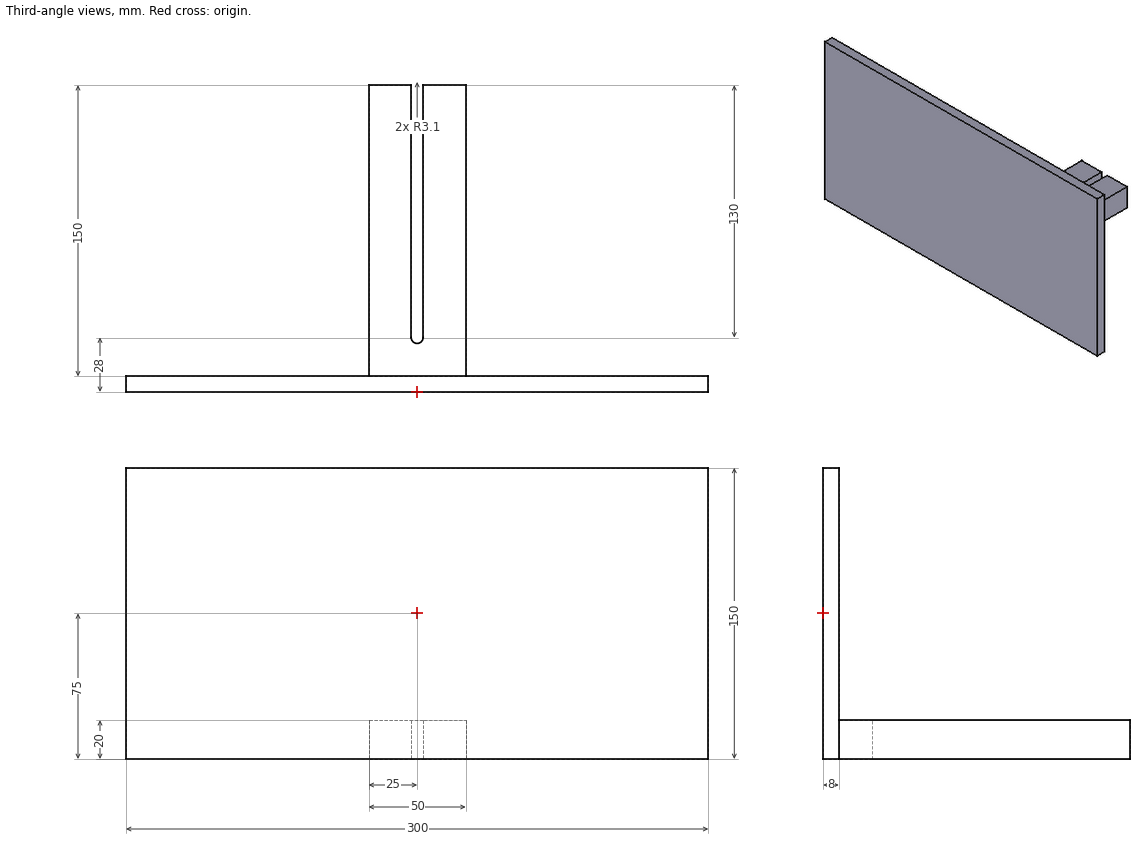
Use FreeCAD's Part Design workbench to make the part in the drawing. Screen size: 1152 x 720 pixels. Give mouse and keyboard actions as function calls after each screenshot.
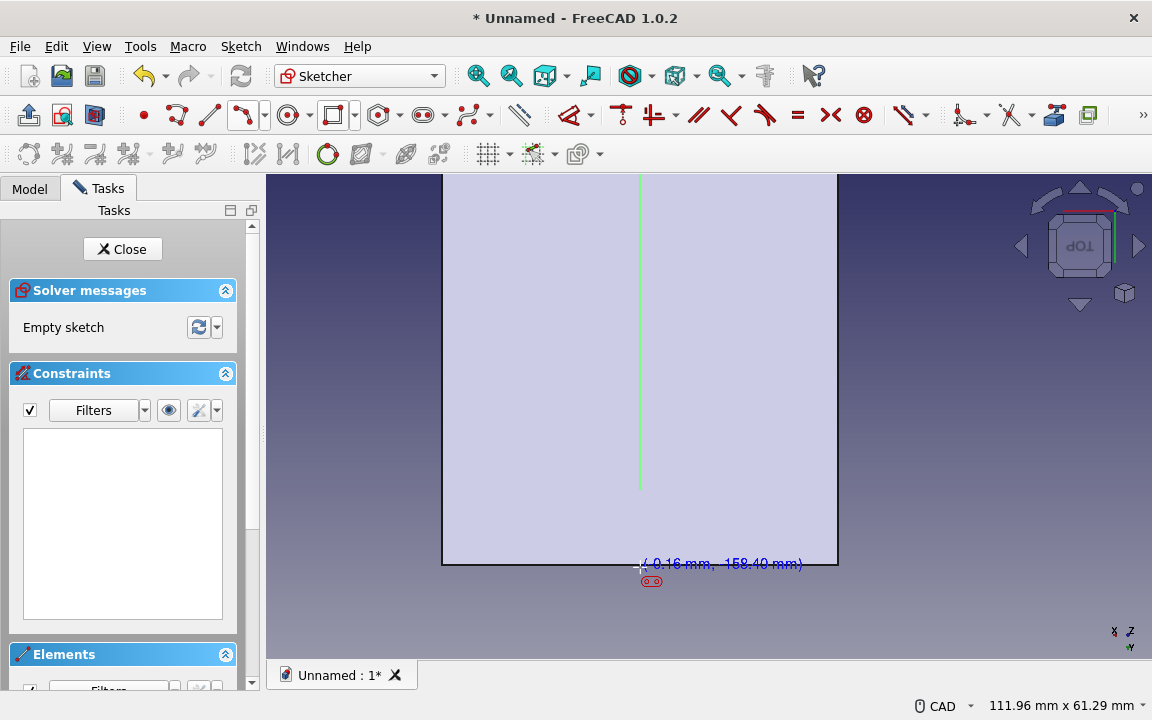
scroll(641, 568, down, 7)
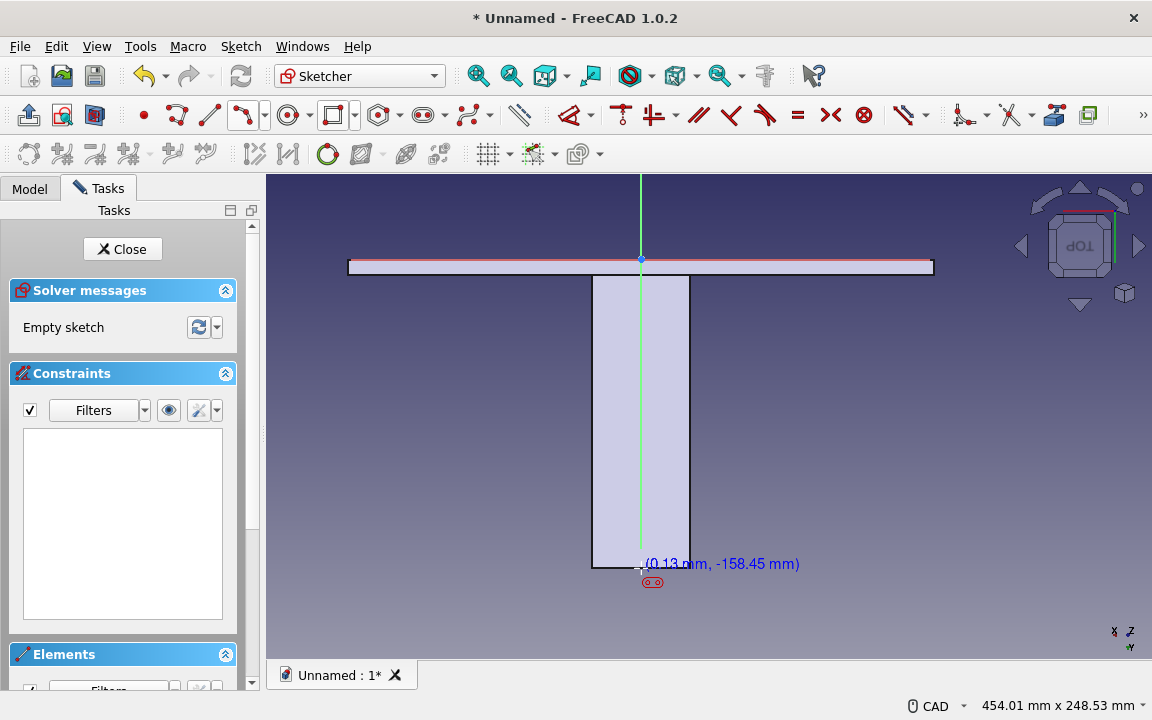
click(641, 568)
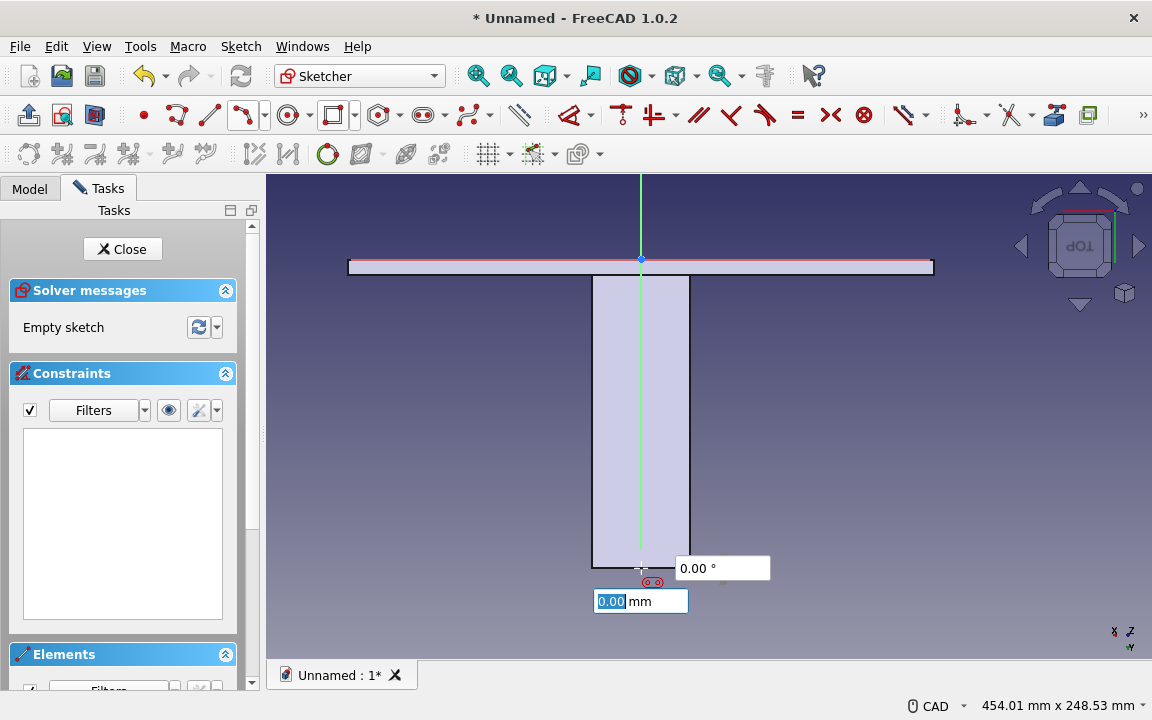
click(650, 314)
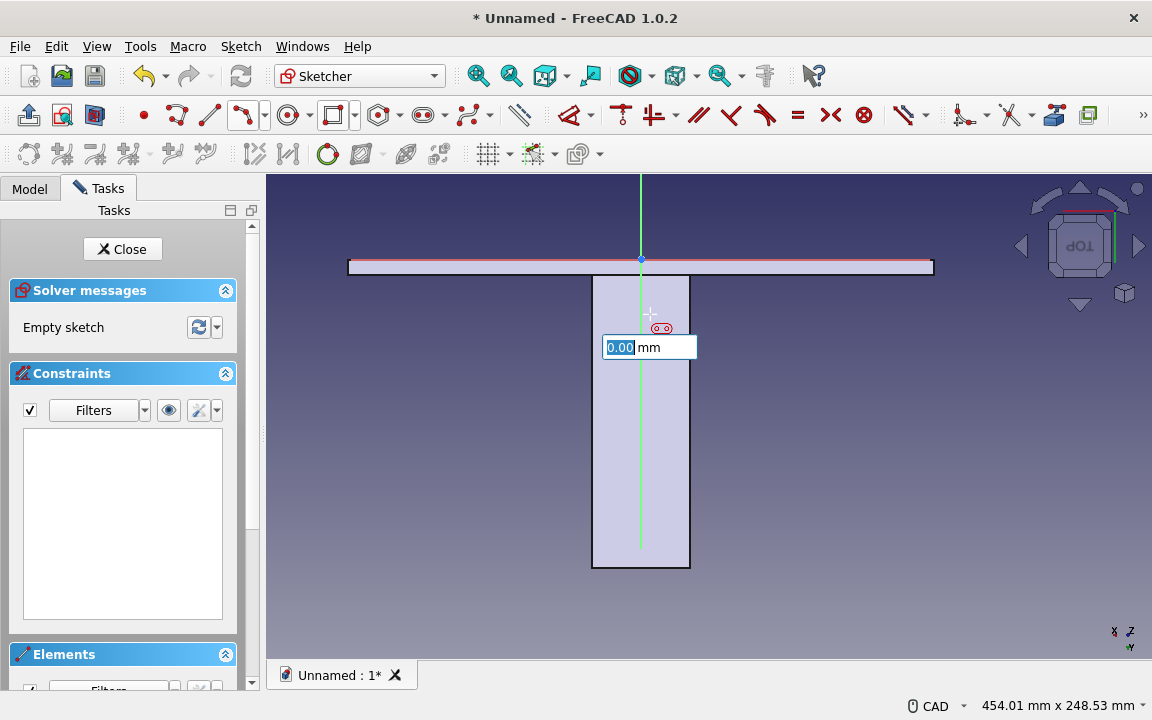
scroll(635, 441, up, 5)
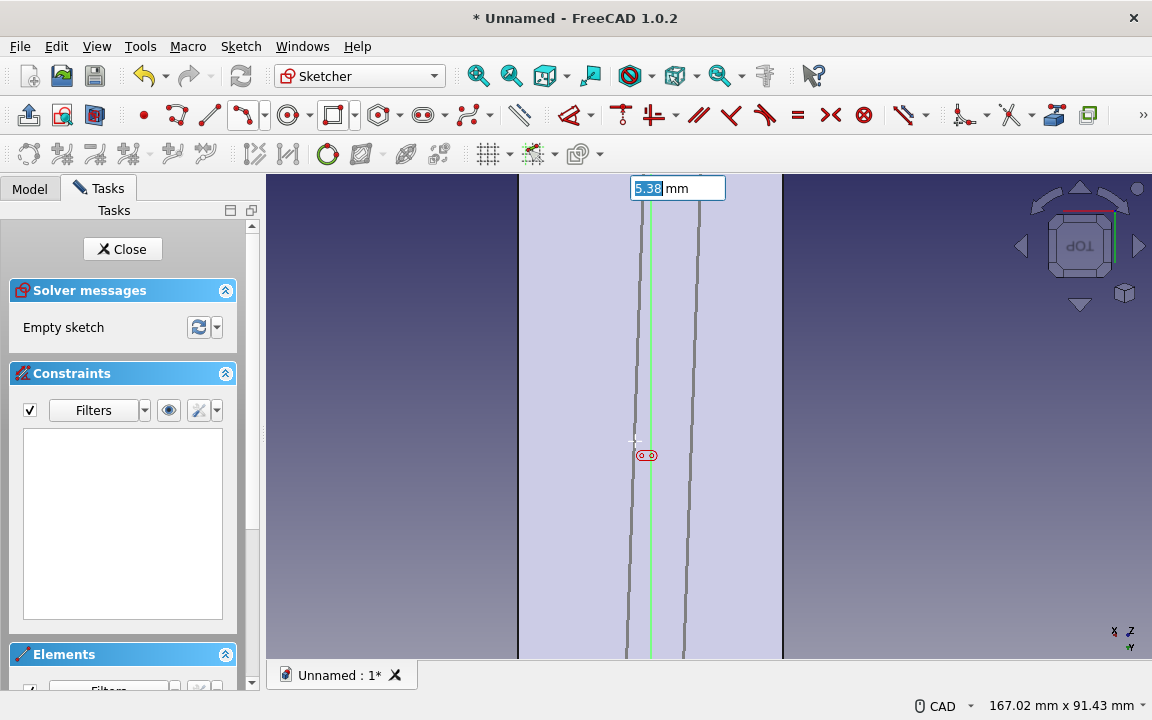
click(634, 440)
key(Escape)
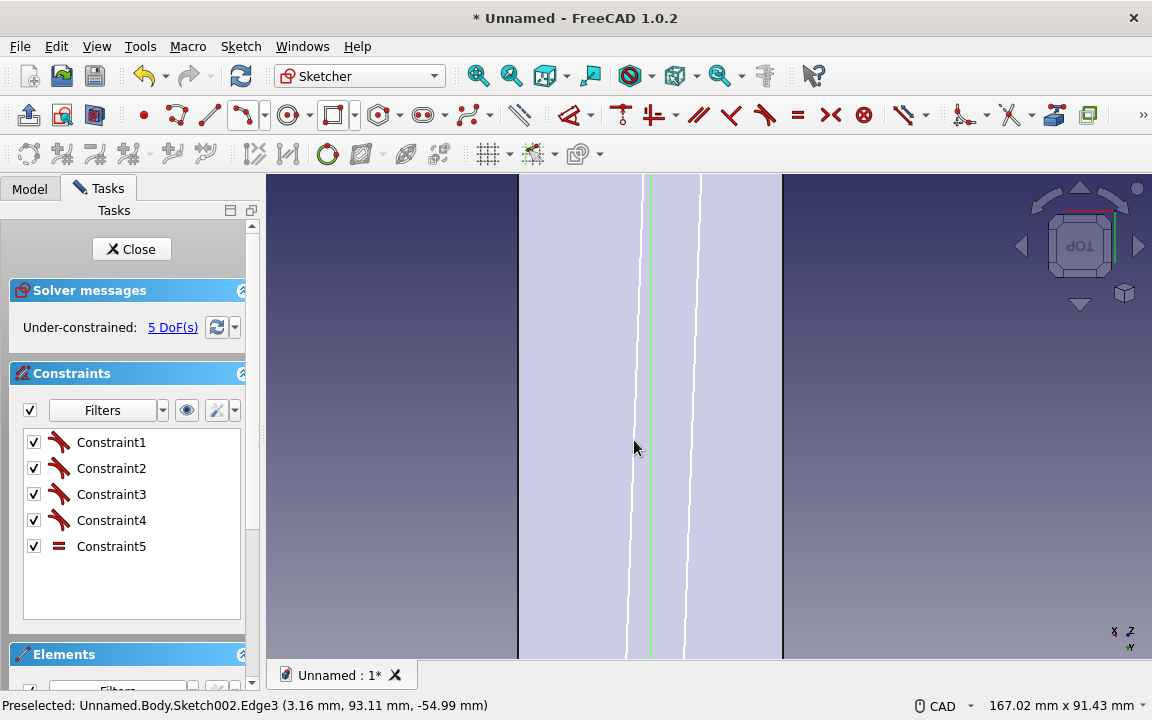
click(629, 580)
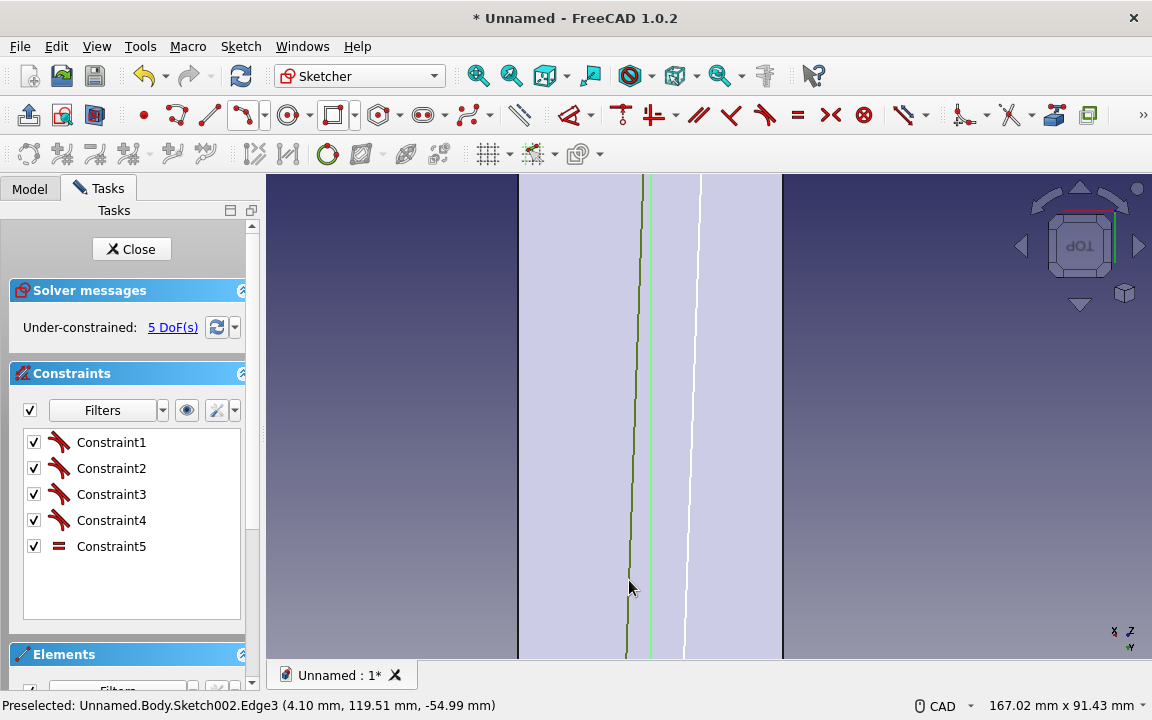
click(676, 116)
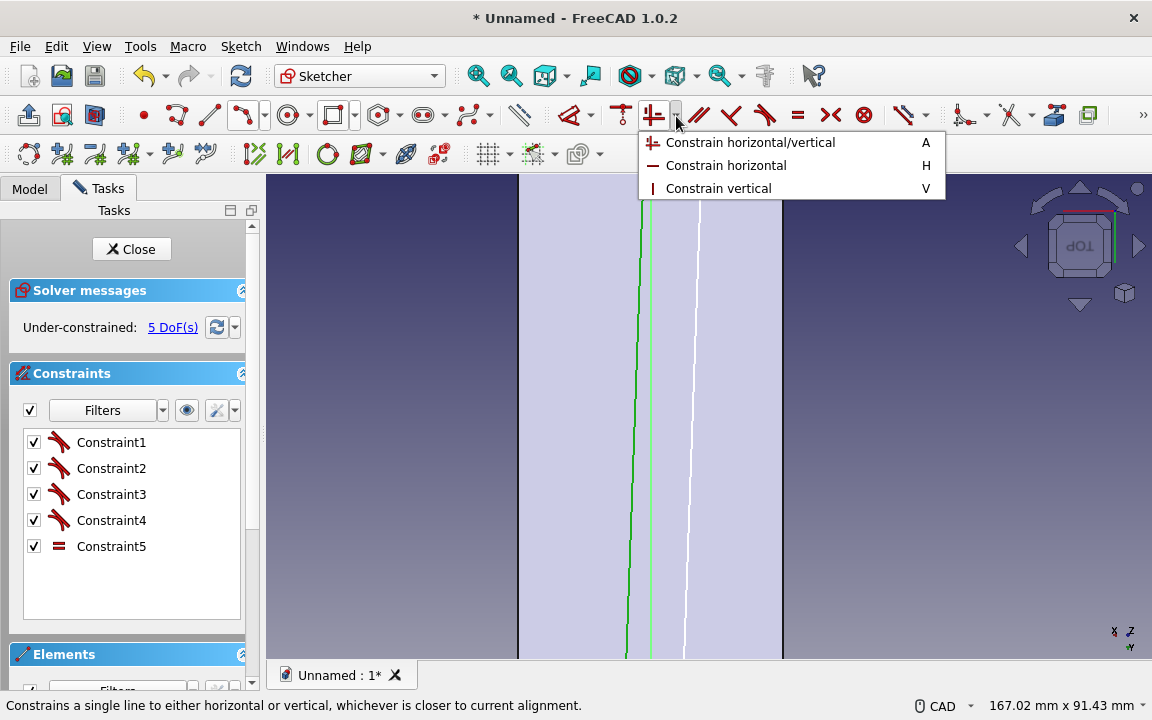
click(792, 188)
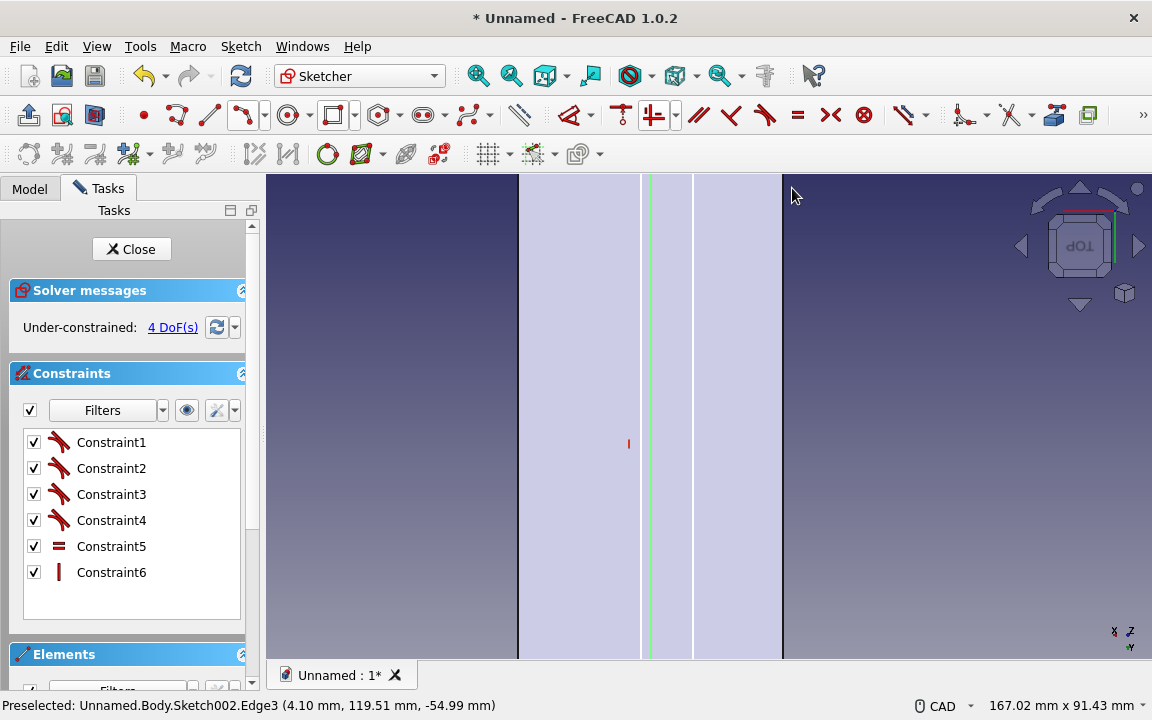
scroll(635, 441, down, 5)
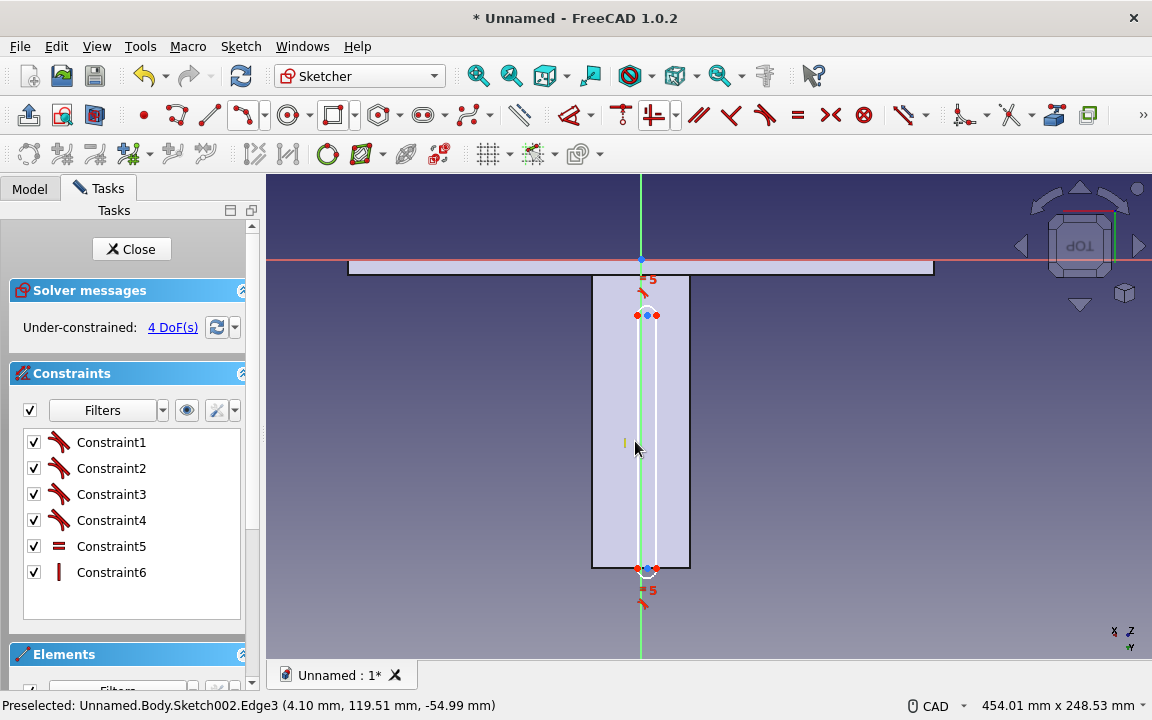
scroll(647, 569, up, 2)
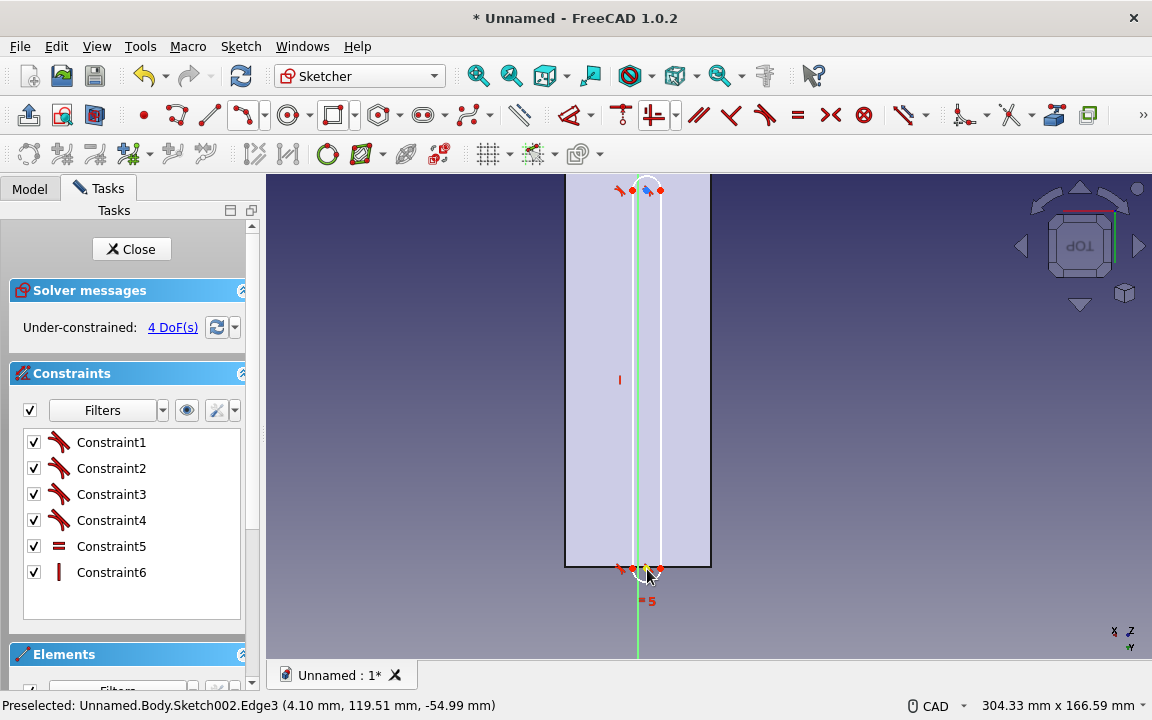
click(647, 568)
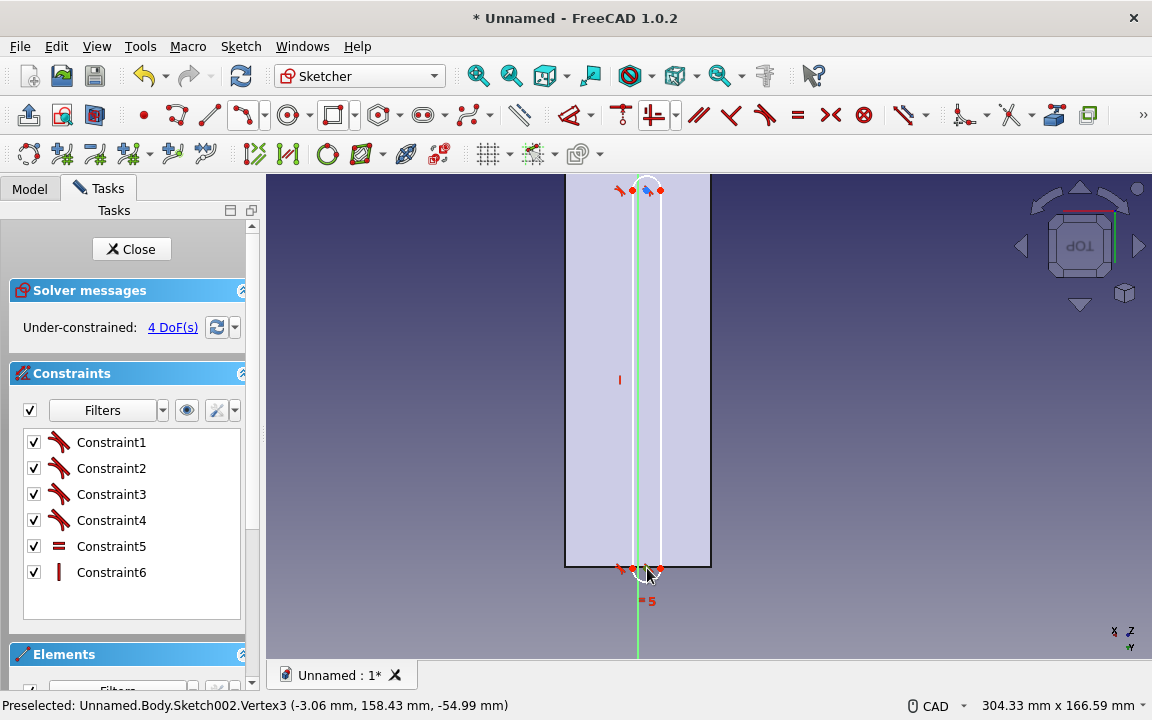
click(638, 539)